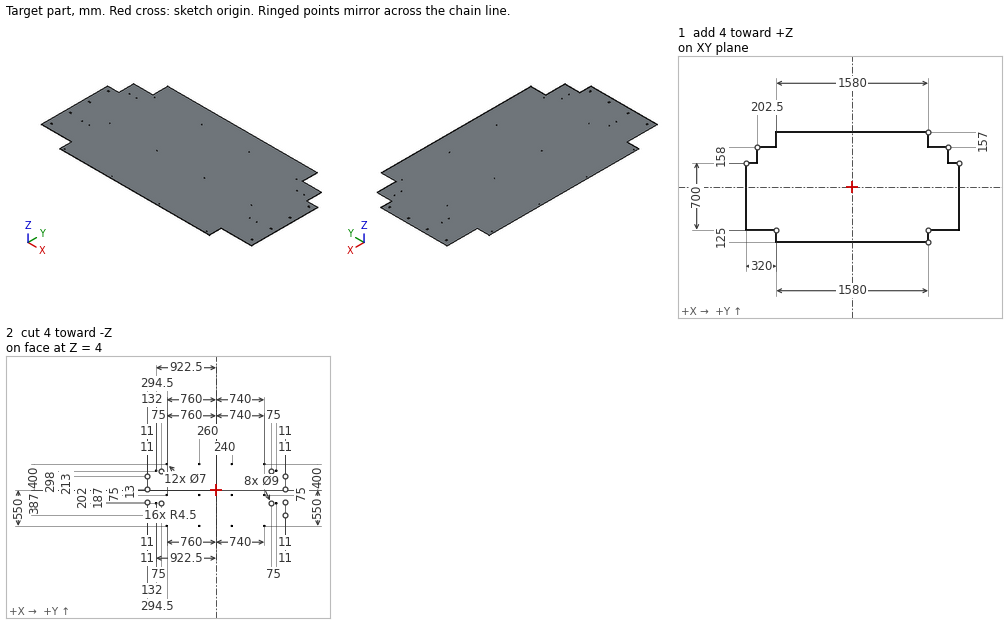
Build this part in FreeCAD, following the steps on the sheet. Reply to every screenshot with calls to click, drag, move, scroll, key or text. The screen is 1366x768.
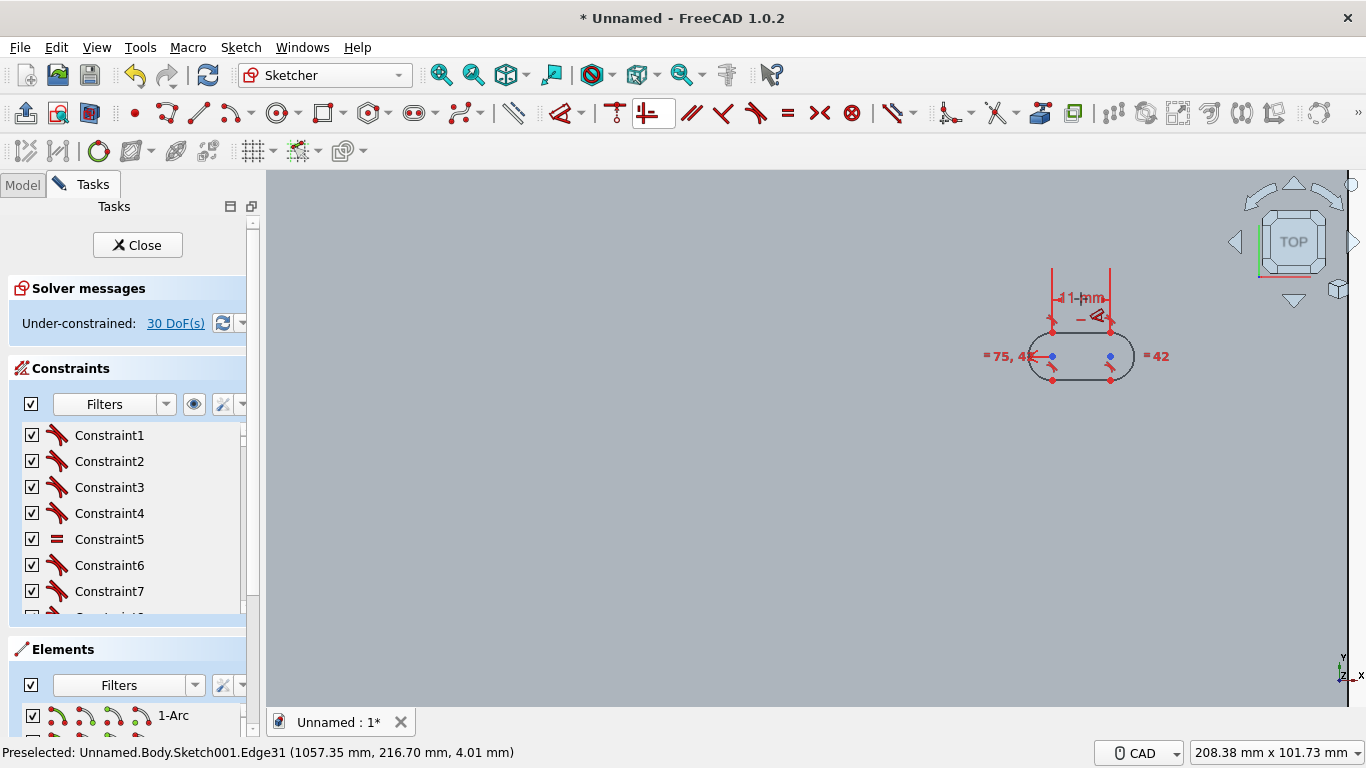
scroll(1088, 346, down, 14)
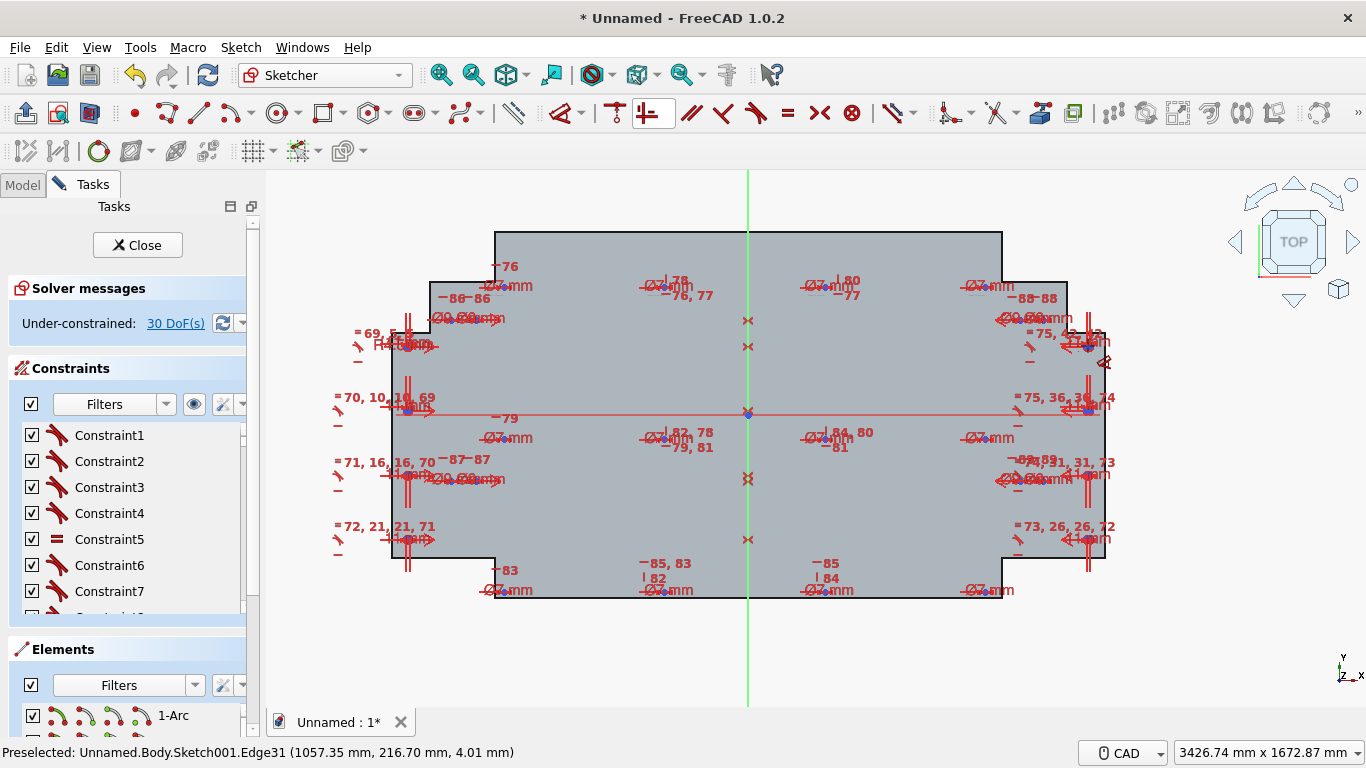
scroll(504, 440, up, 3)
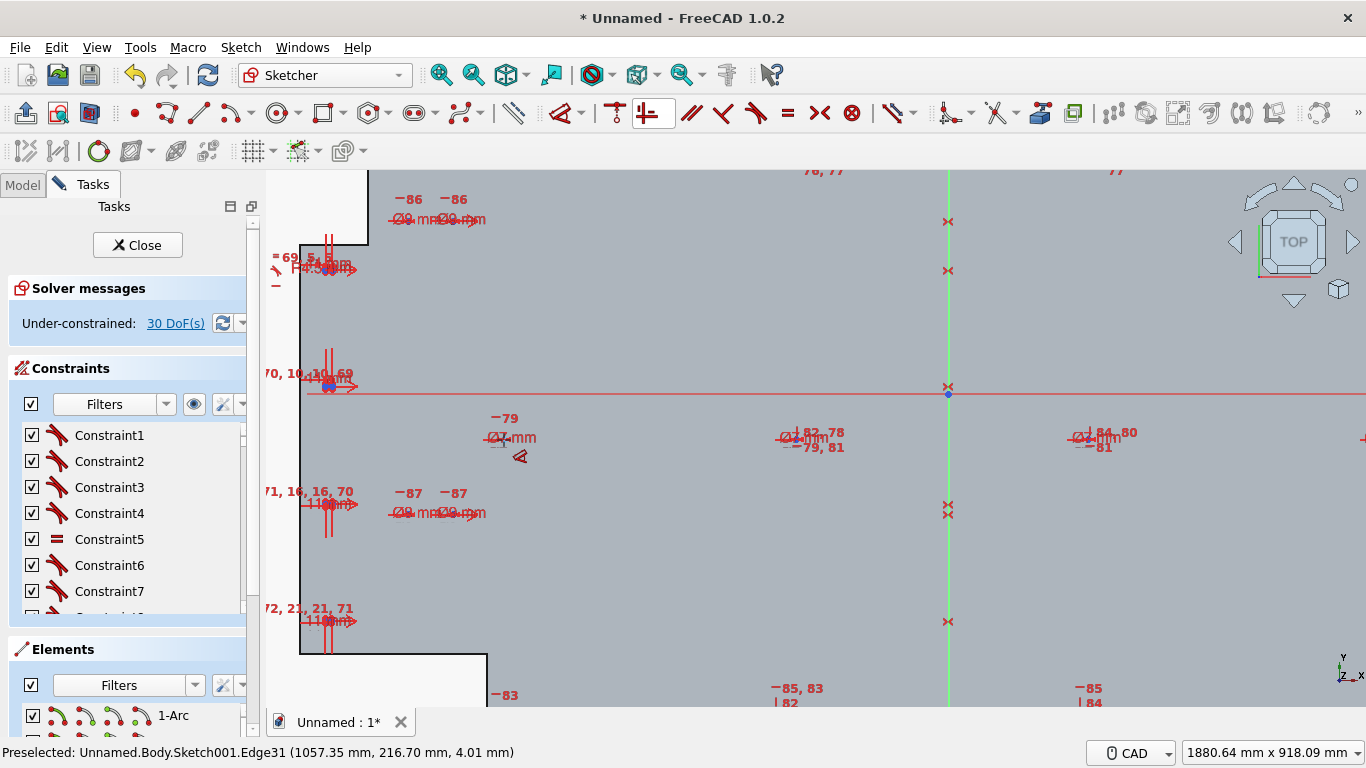
click(504, 440)
click(470, 417)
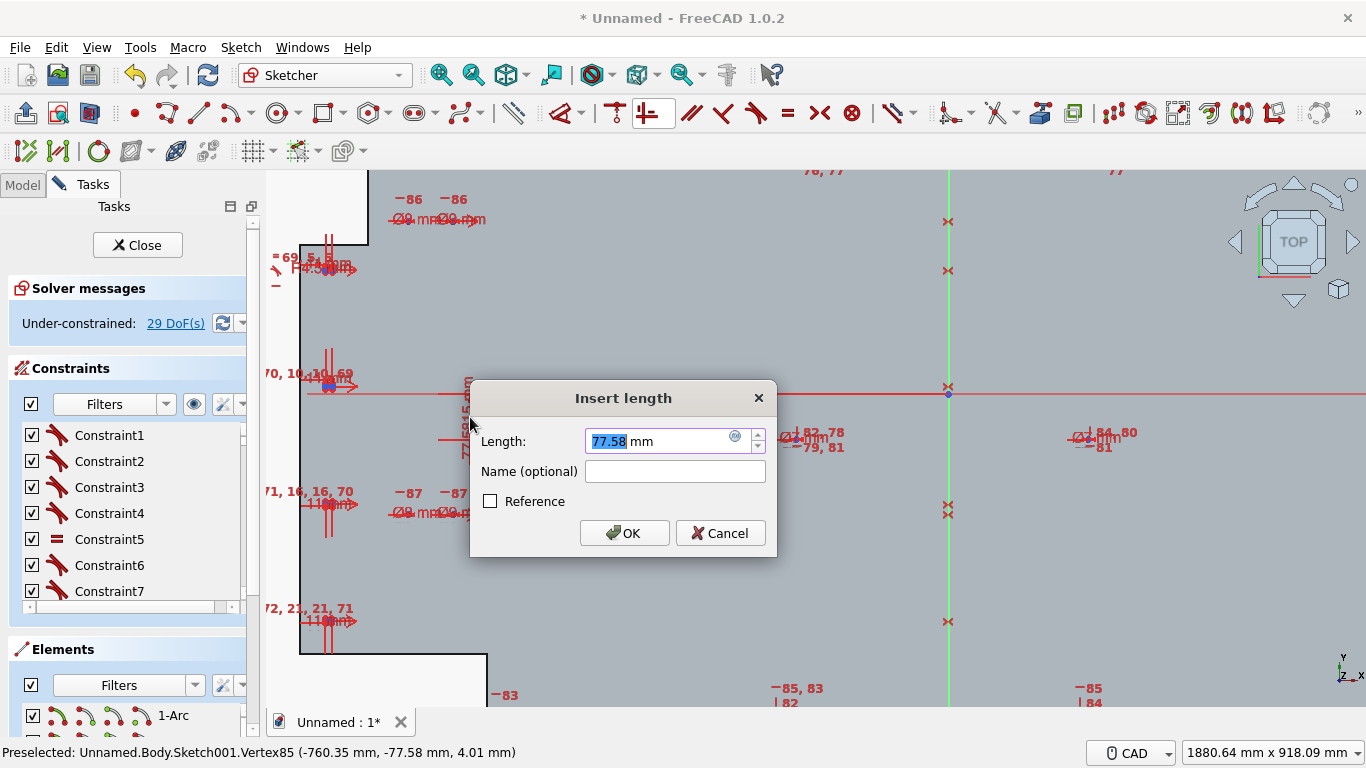
text(75)
key(Return)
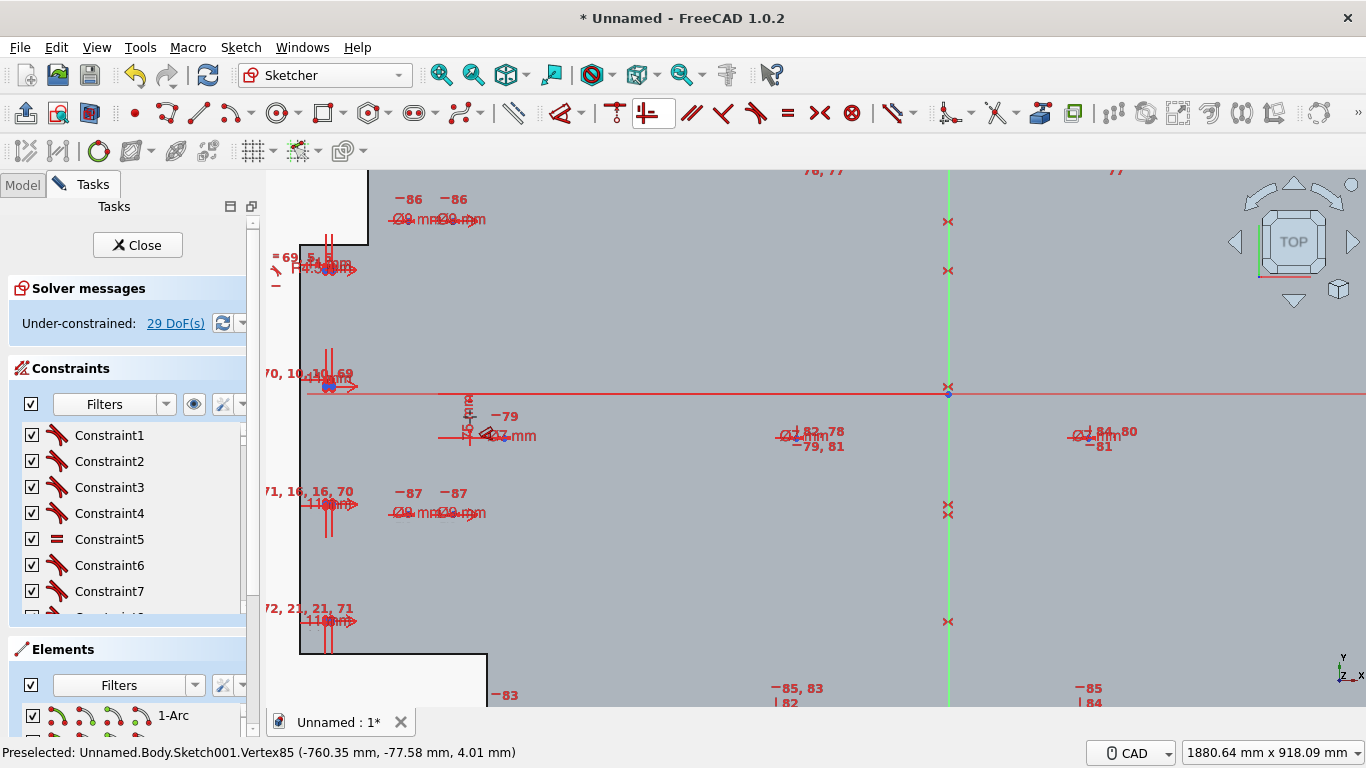
scroll(503, 439, down, 3)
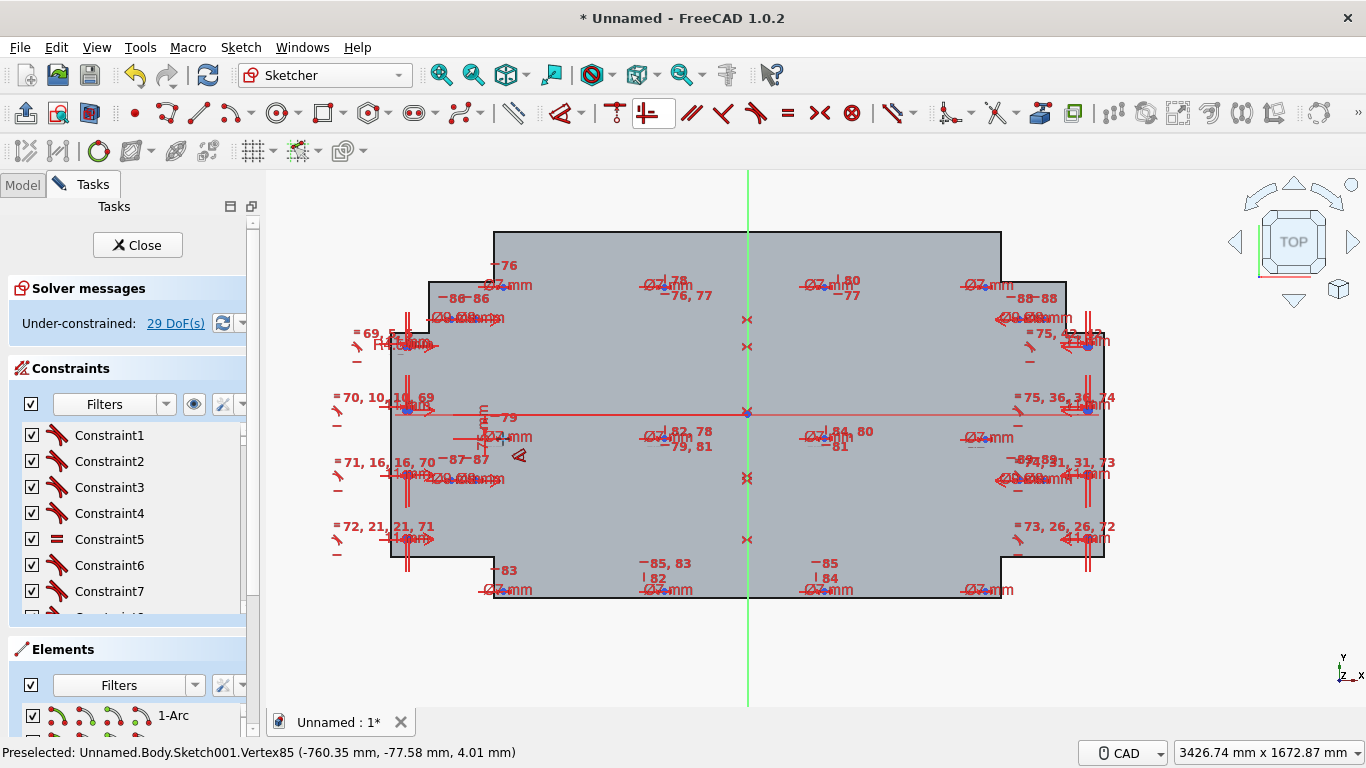
scroll(985, 440, up, 3)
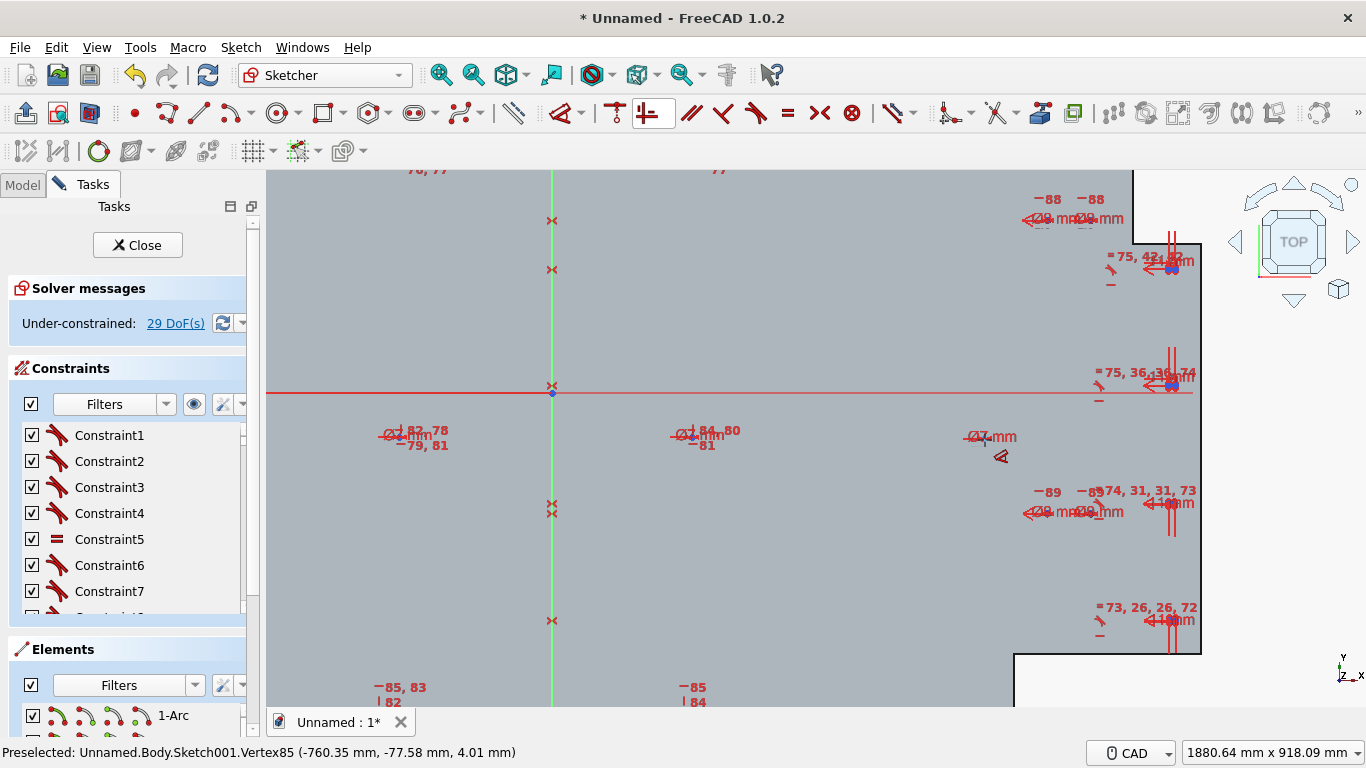
click(985, 439)
click(1019, 416)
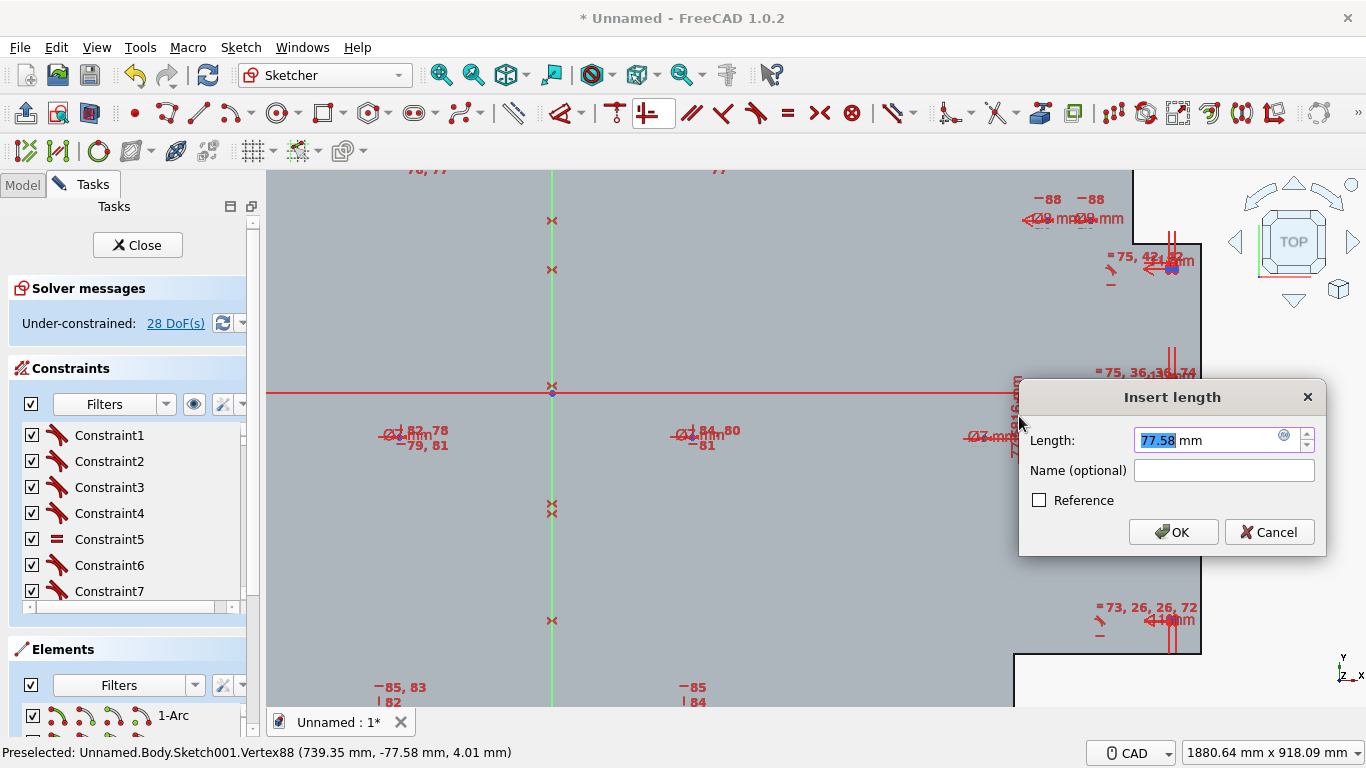
text(75)
key(Return)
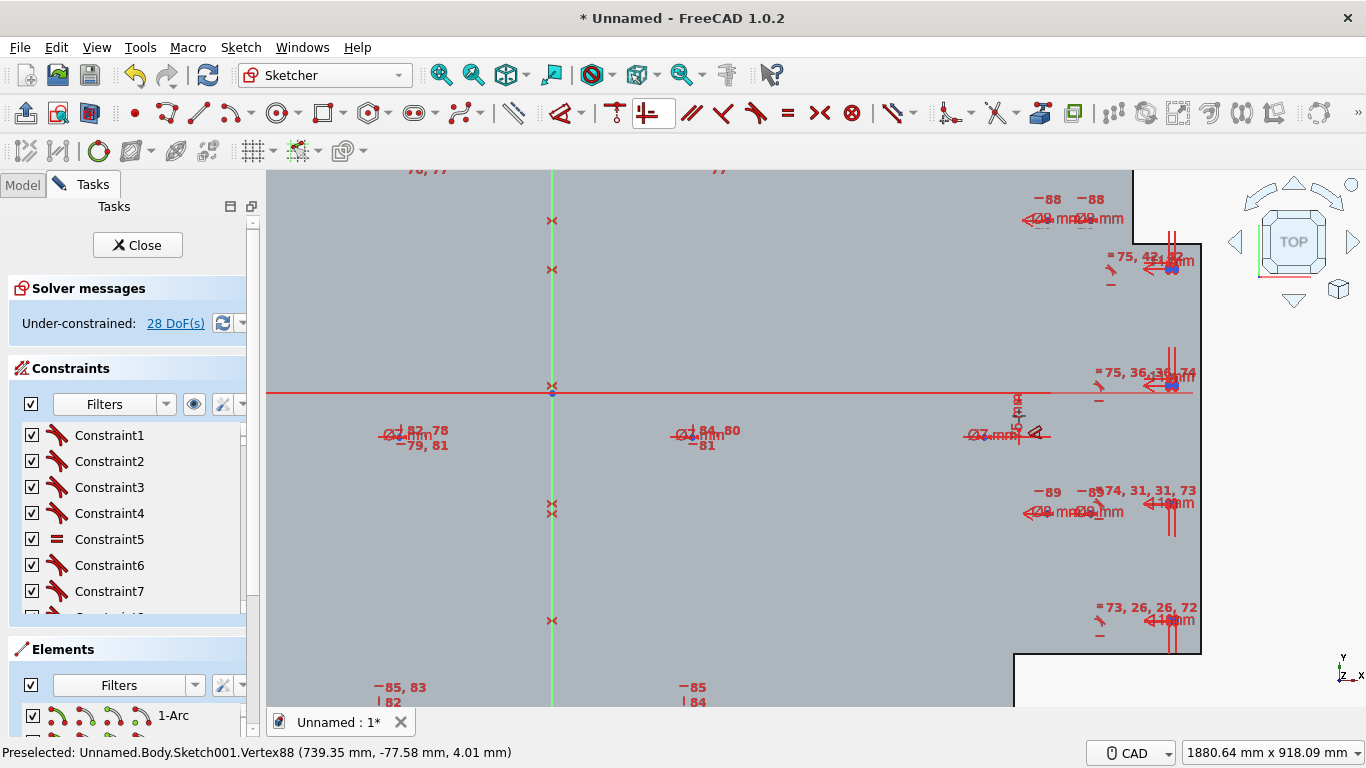
scroll(985, 440, down, 3)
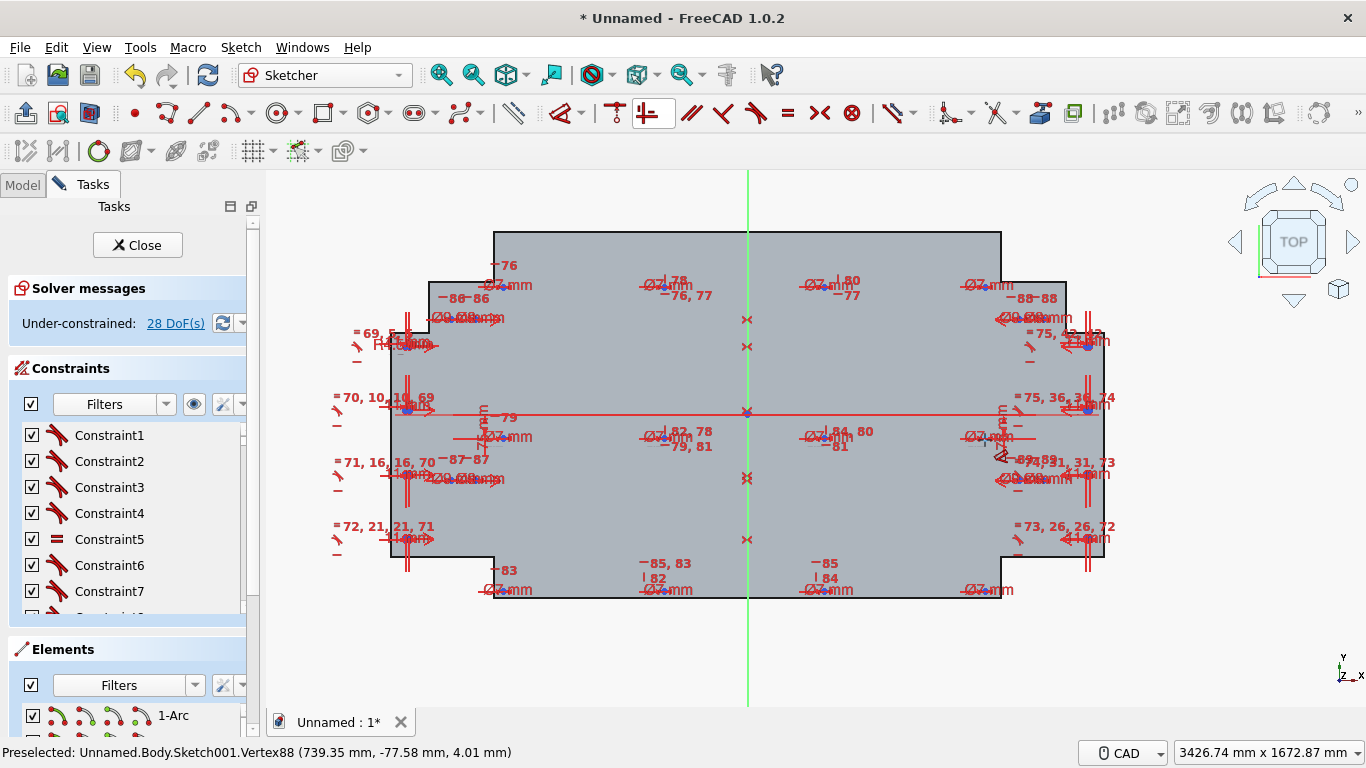
scroll(406, 410, up, 12)